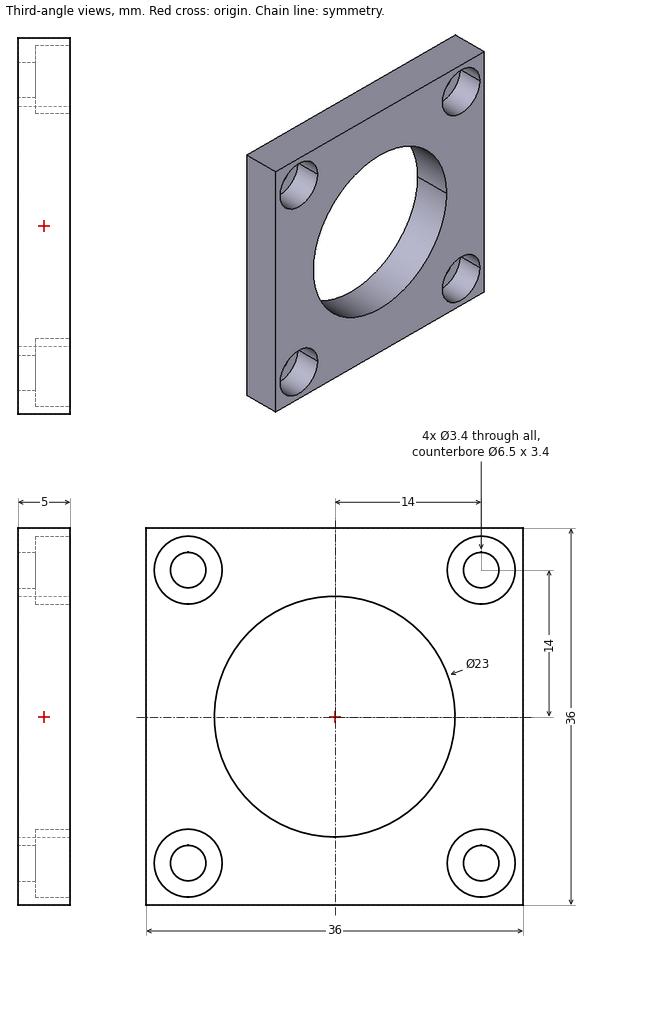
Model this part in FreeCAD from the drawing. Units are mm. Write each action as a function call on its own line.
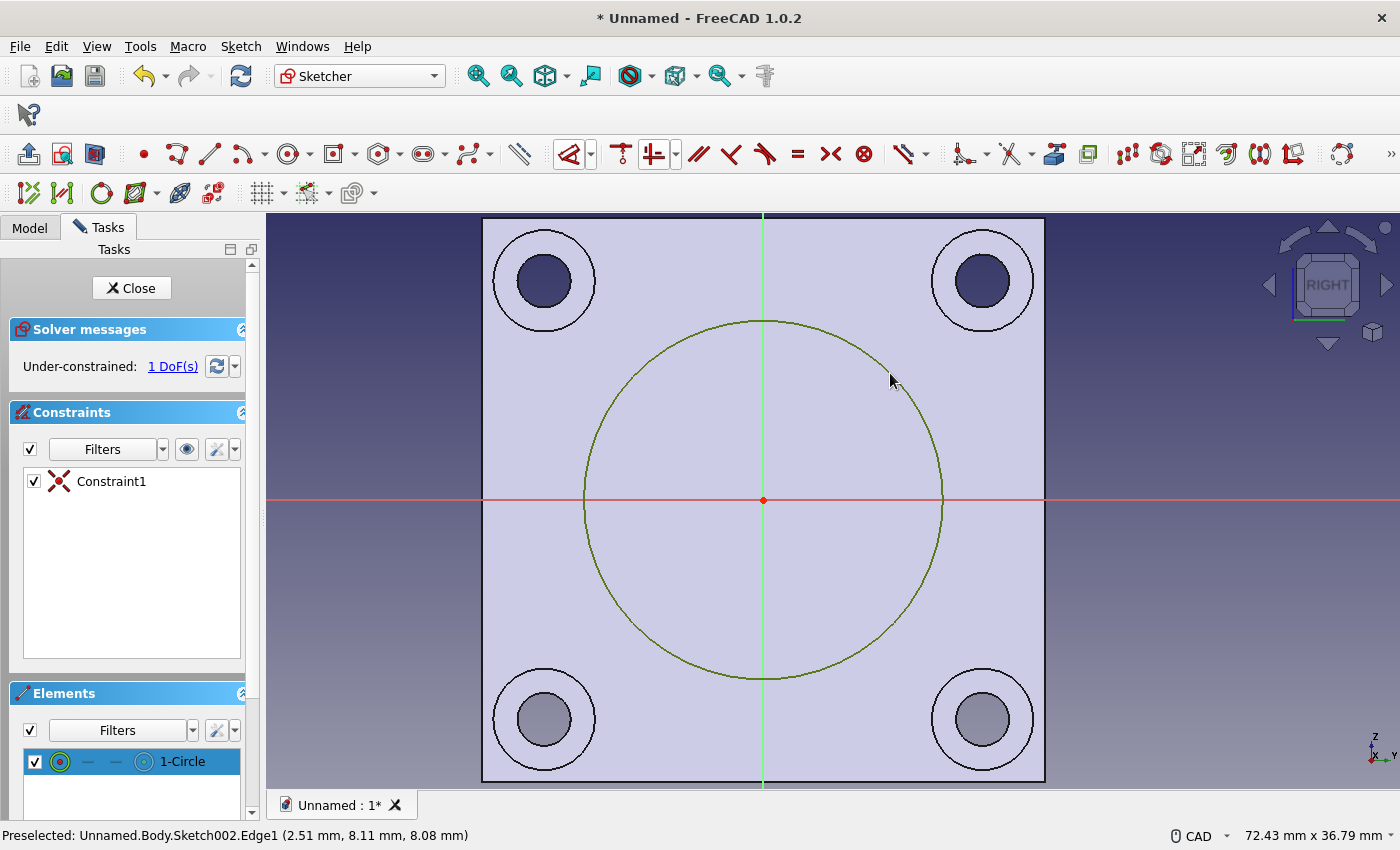
click(590, 154)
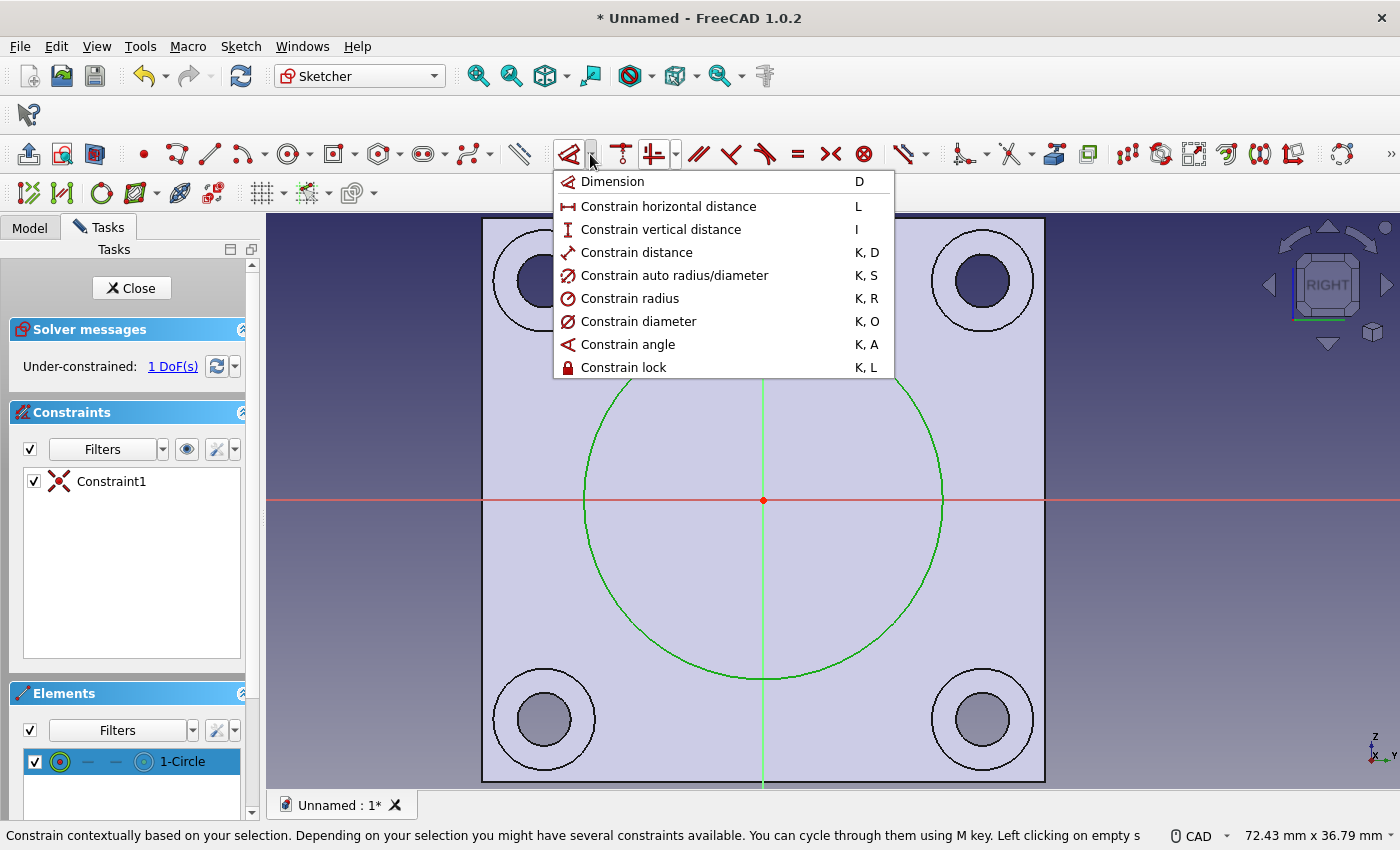
click(724, 322)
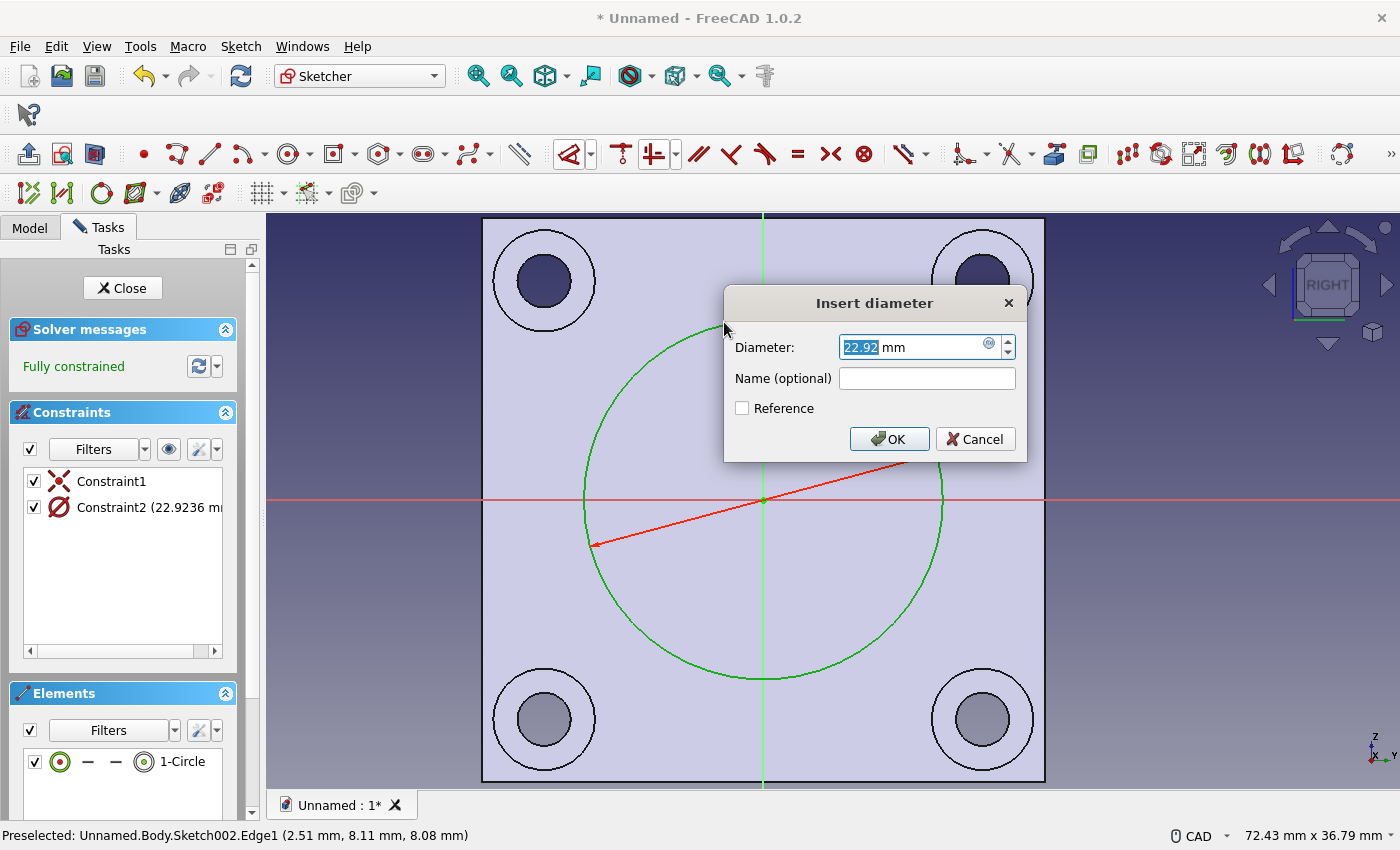
text(23)
key(Return)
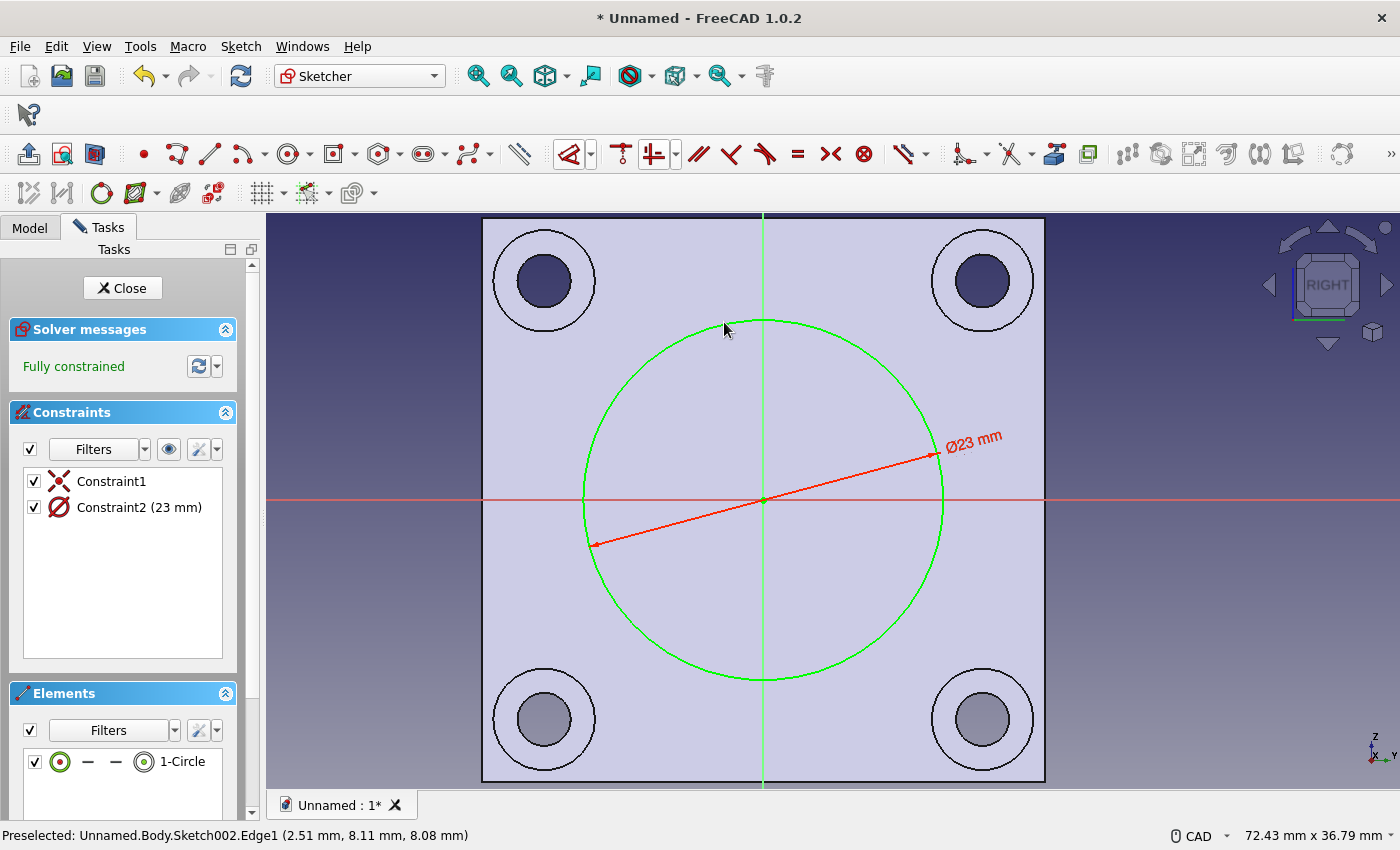
click(123, 288)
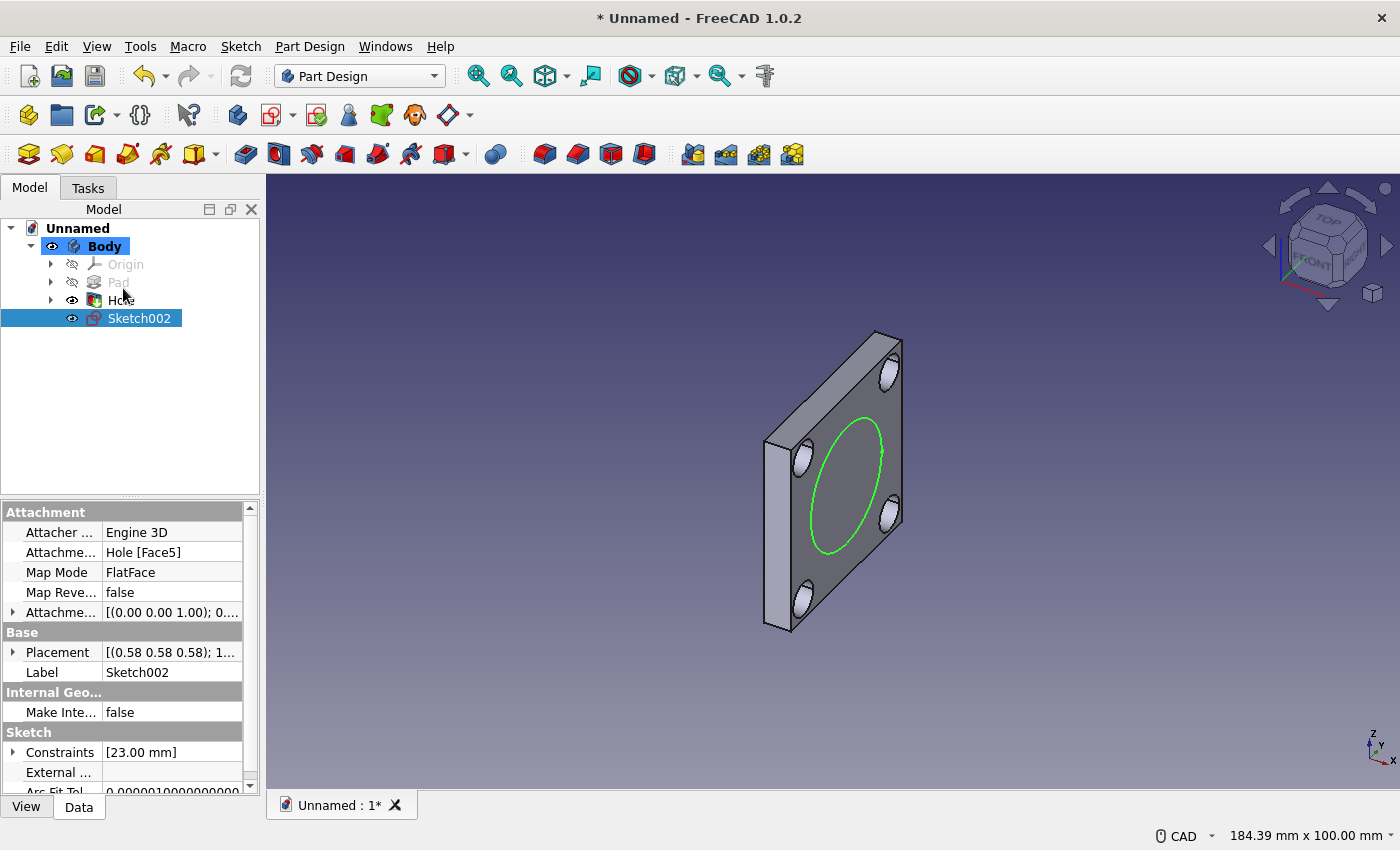
click(246, 154)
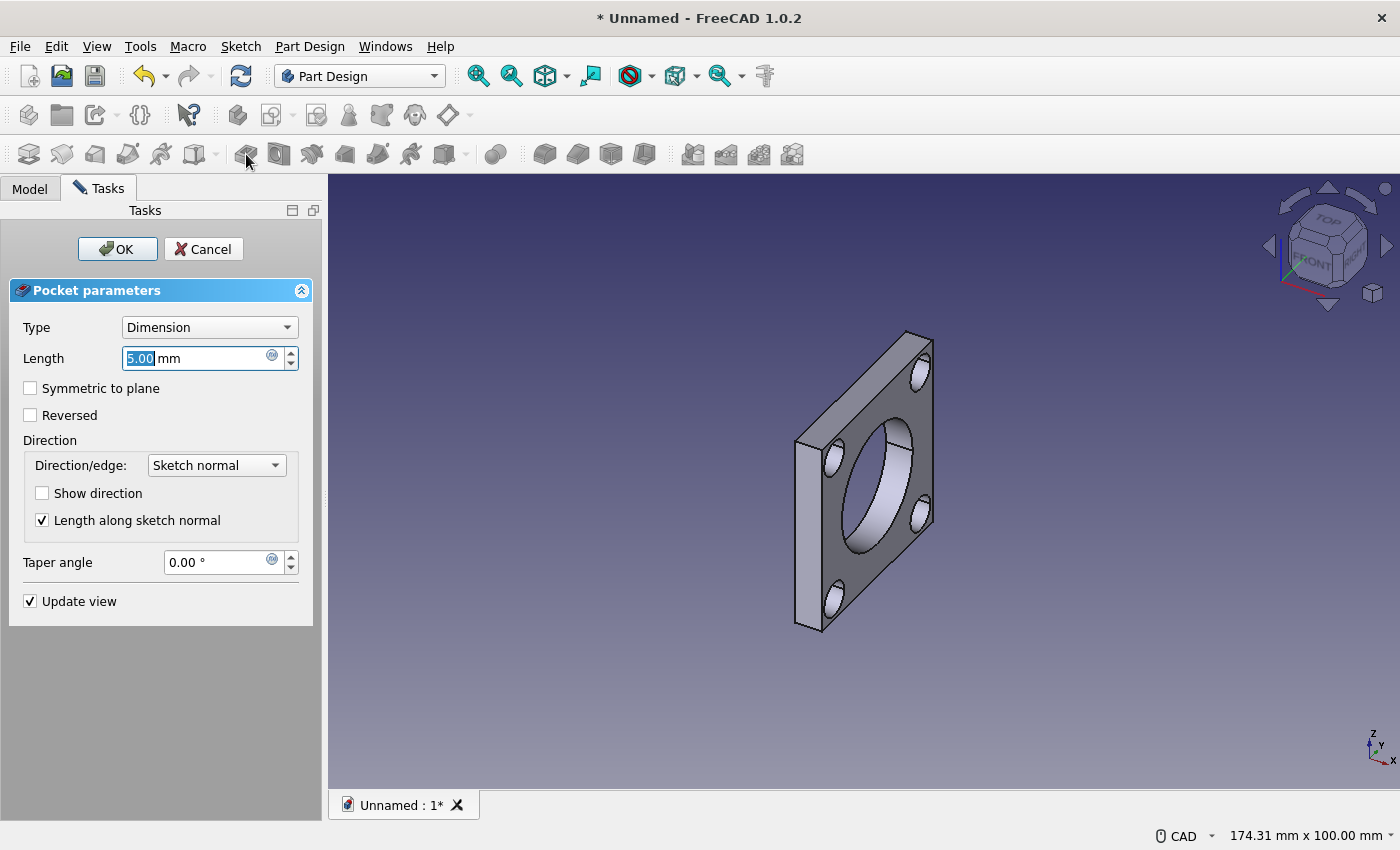
click(210, 328)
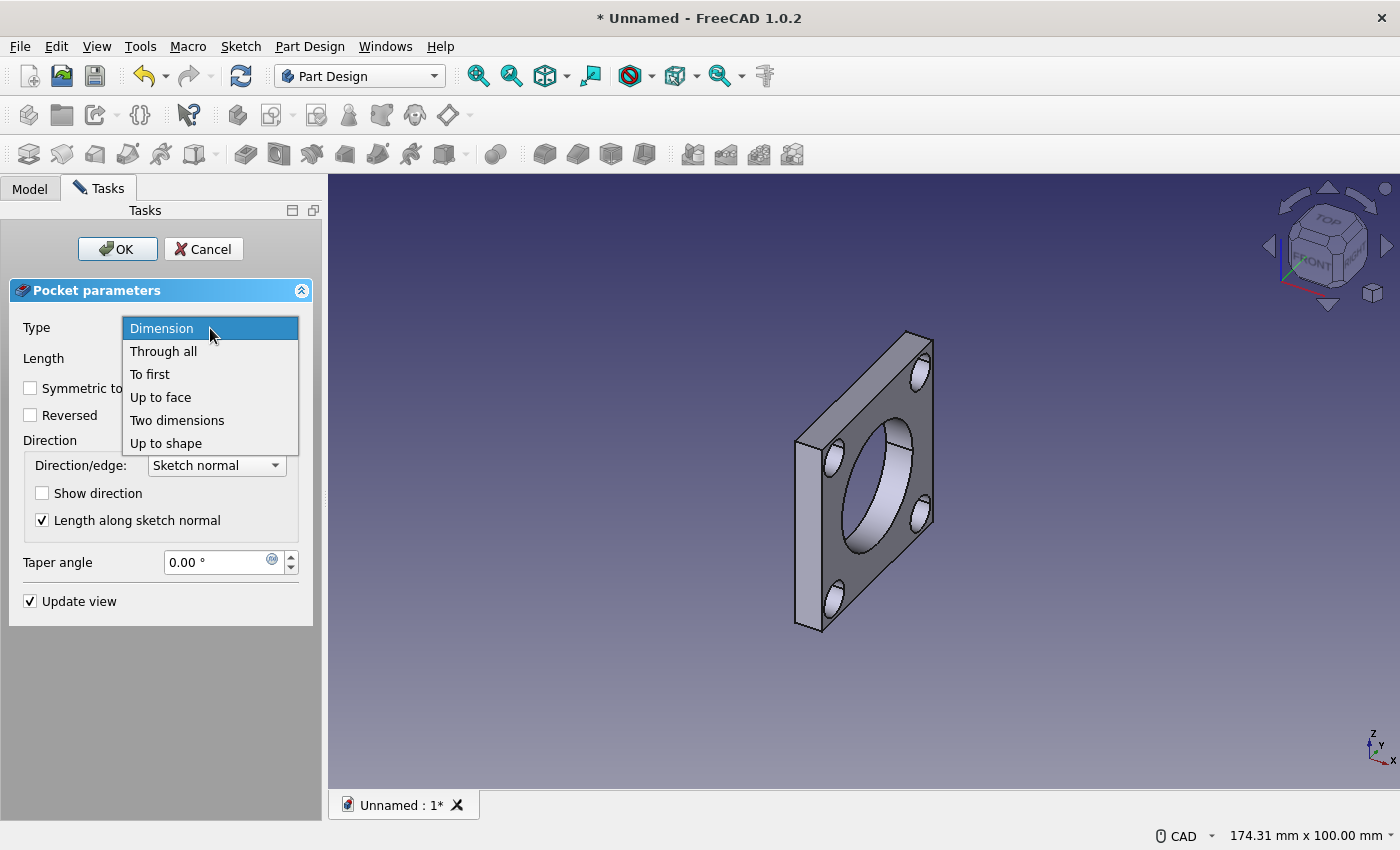
click(208, 352)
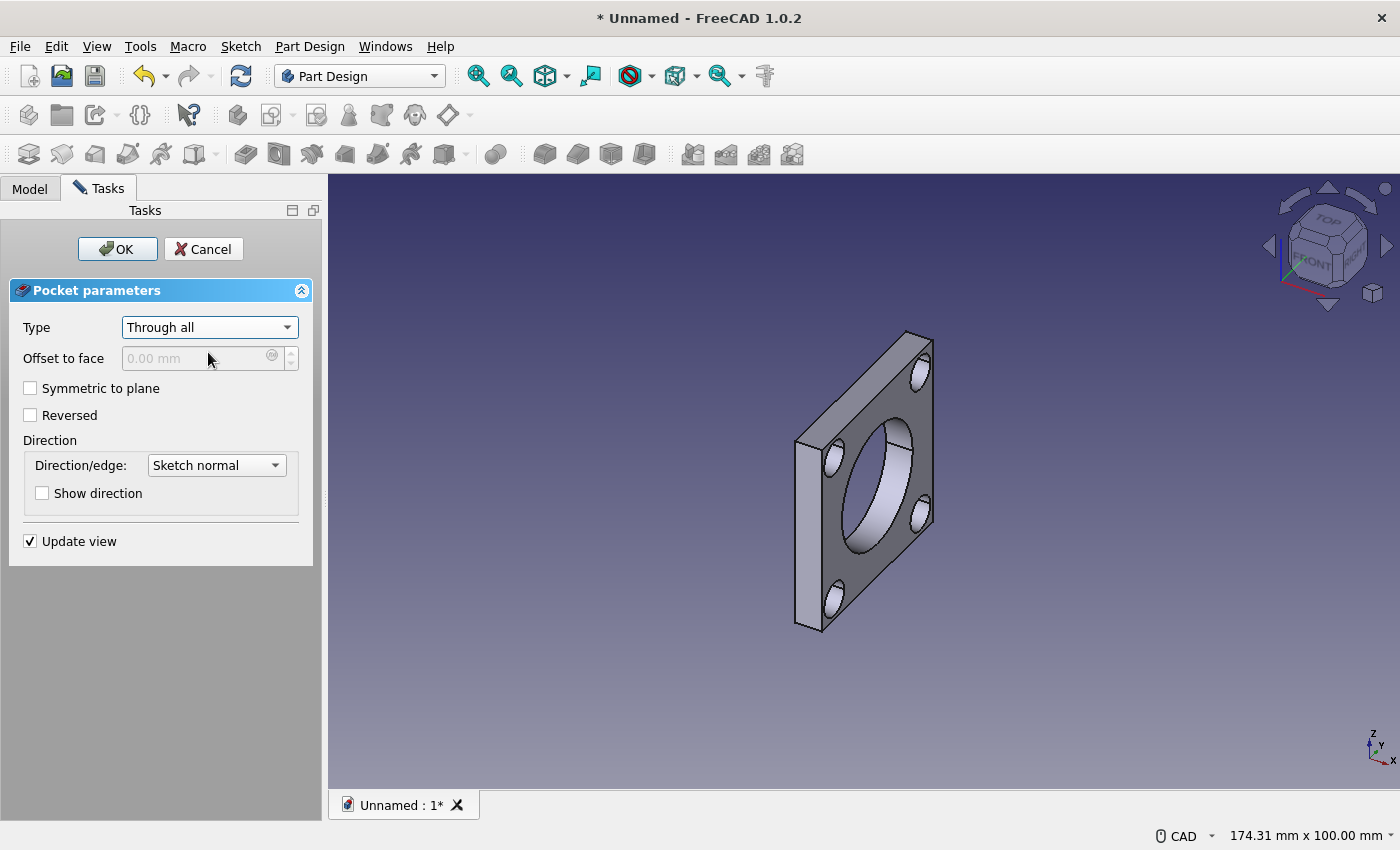
click(118, 249)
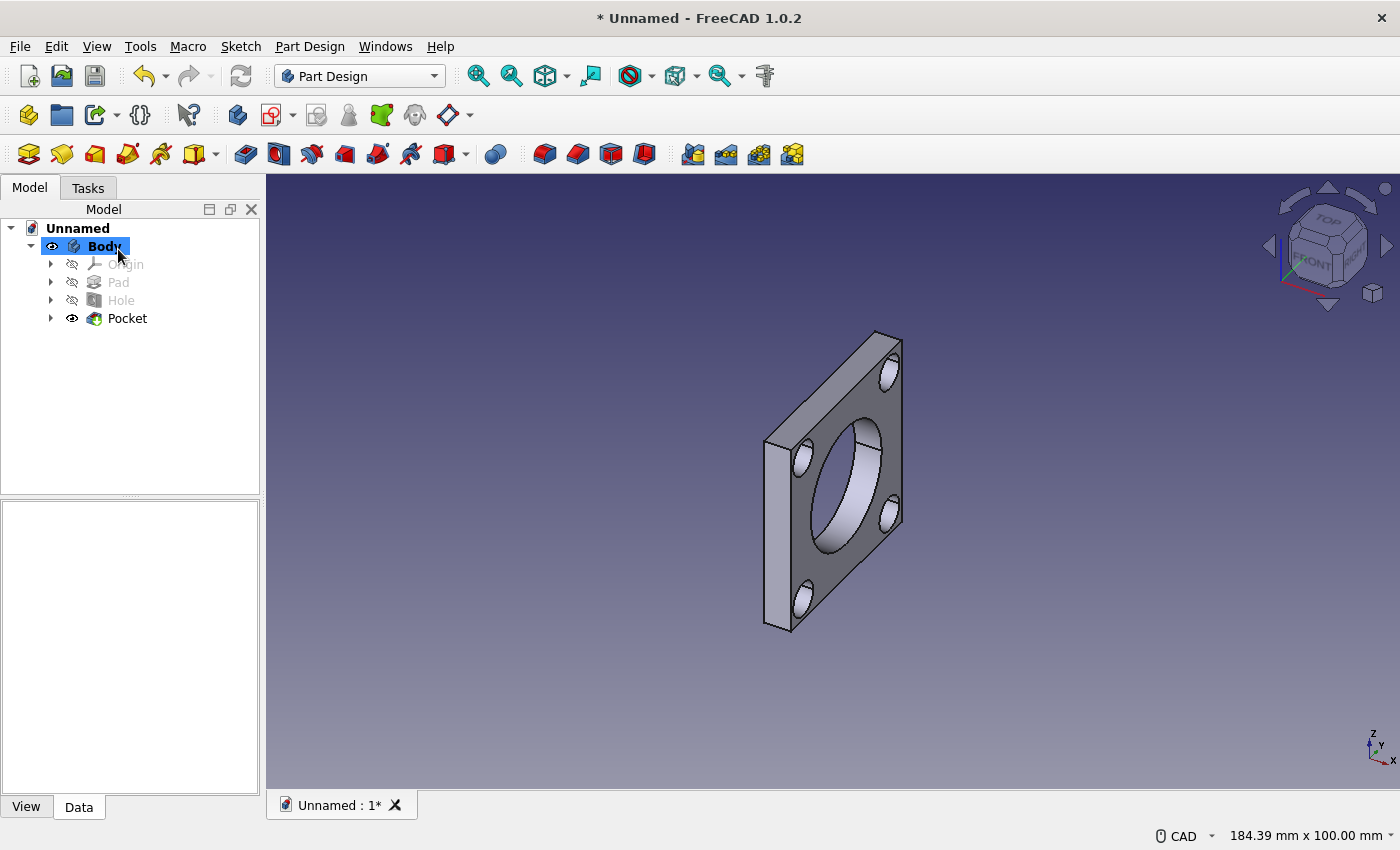
key(0)